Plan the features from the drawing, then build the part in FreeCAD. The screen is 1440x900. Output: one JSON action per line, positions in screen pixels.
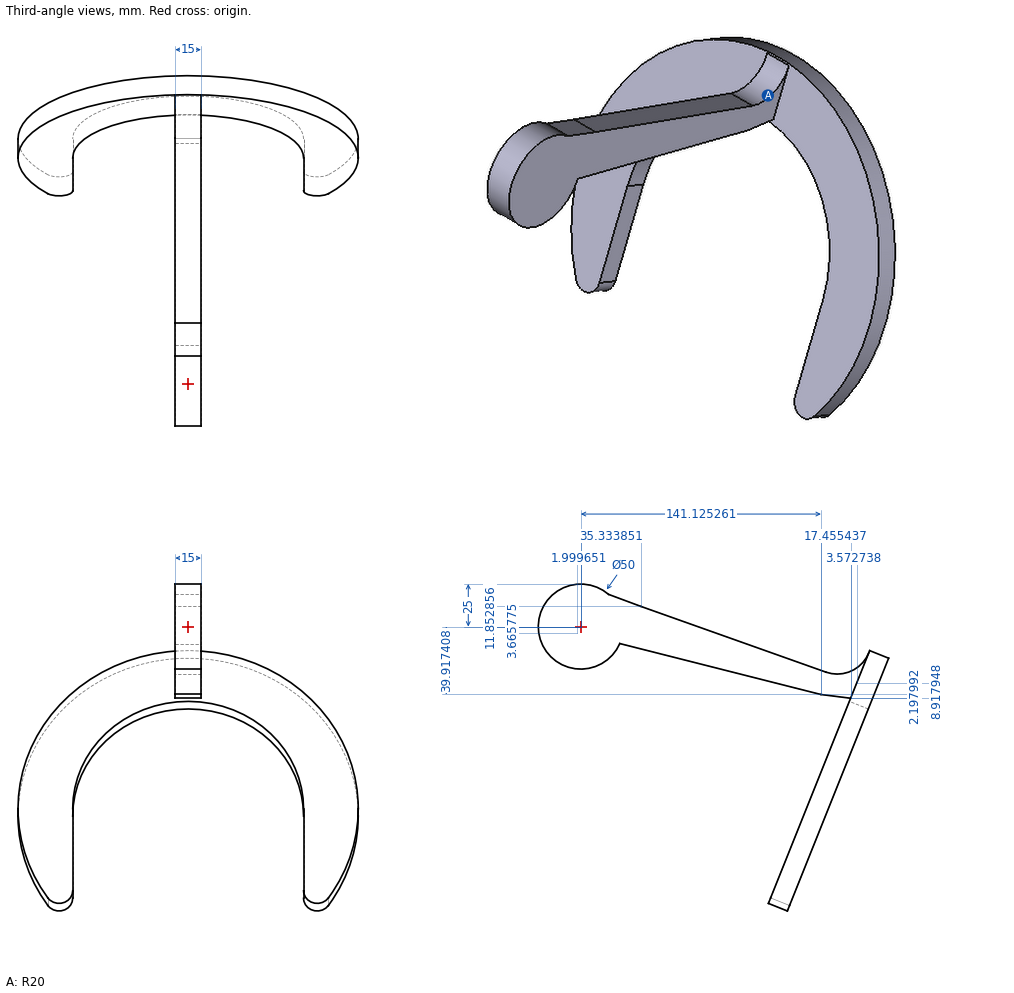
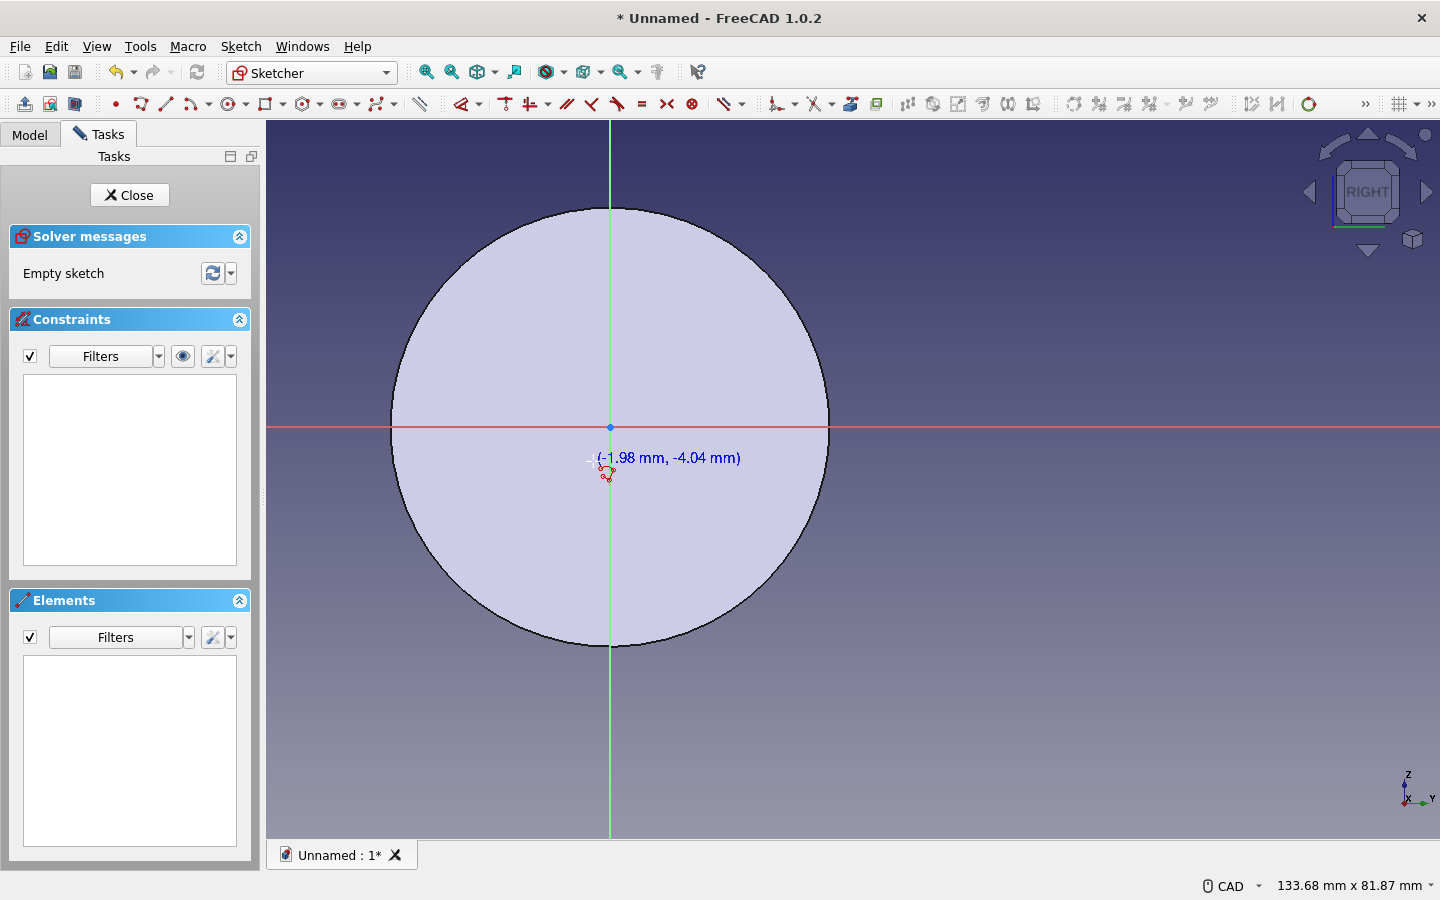
{"action": "left_click", "coordinate": [592, 459]}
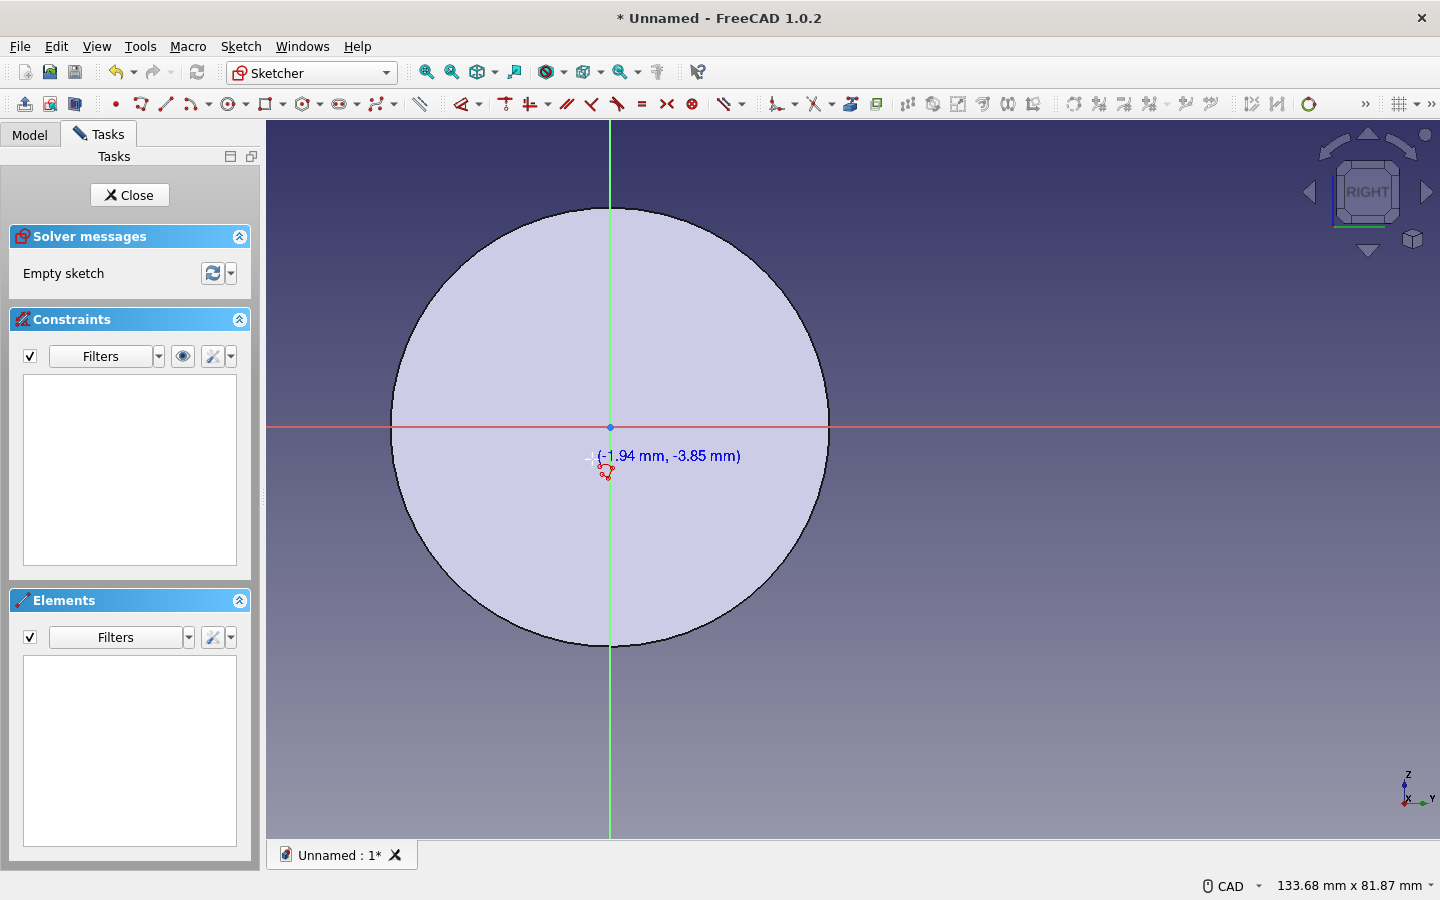
{"action": "scroll", "coordinate": [353, 461], "scroll_direction": "down", "scroll_amount": 4}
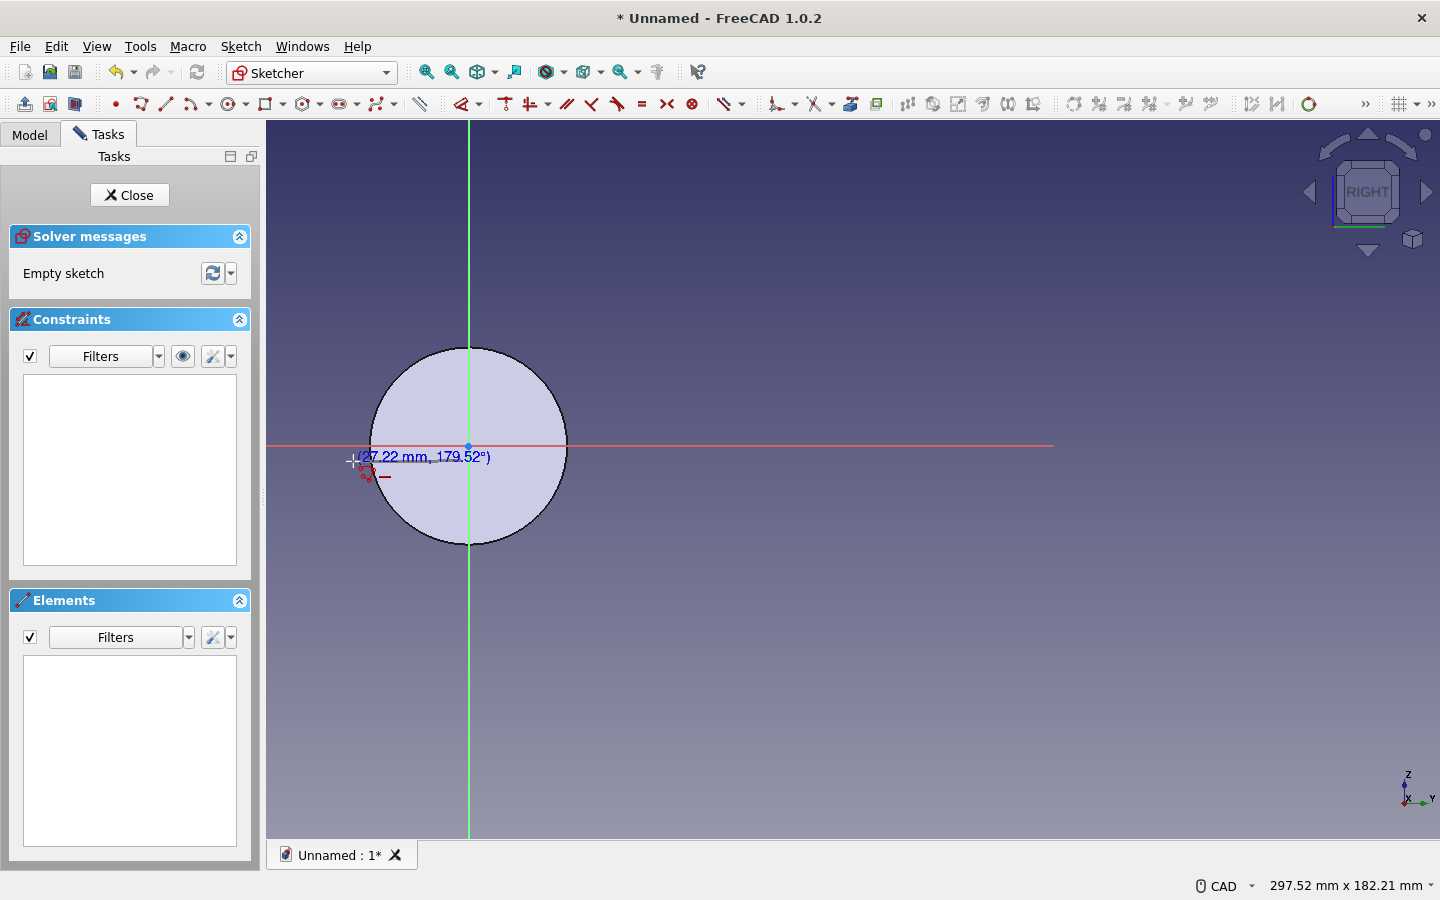
{"action": "left_click", "coordinate": [1025, 604]}
{"action": "left_click", "coordinate": [1094, 612]}
{"action": "left_click", "coordinate": [1108, 577]}
{"action": "left_click", "coordinate": [608, 399]}
{"action": "left_click", "coordinate": [469, 347]}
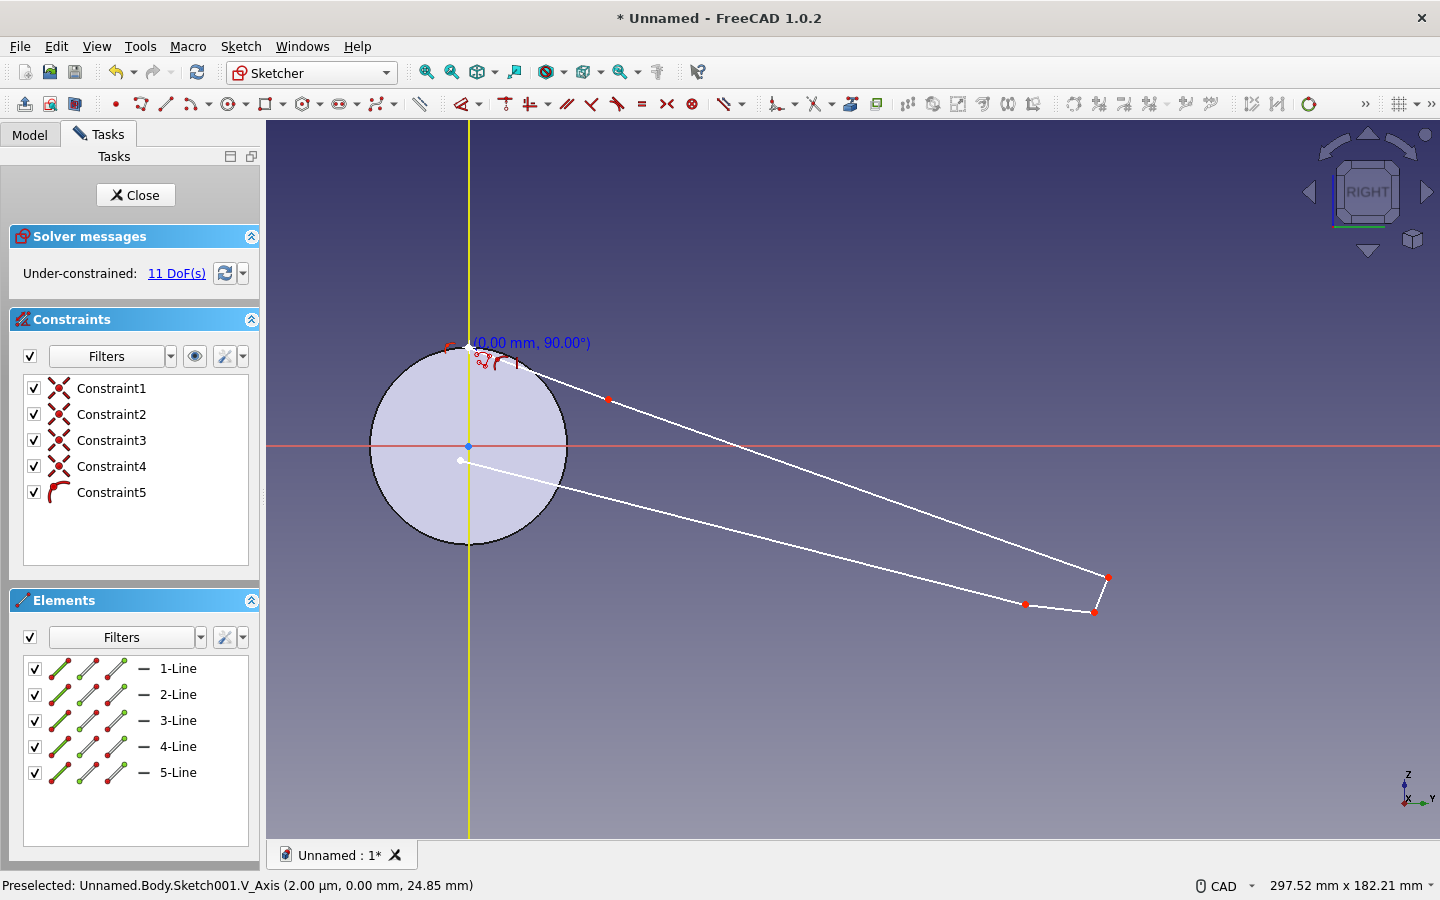
{"action": "scroll", "coordinate": [461, 461], "scroll_direction": "up", "scroll_amount": 4}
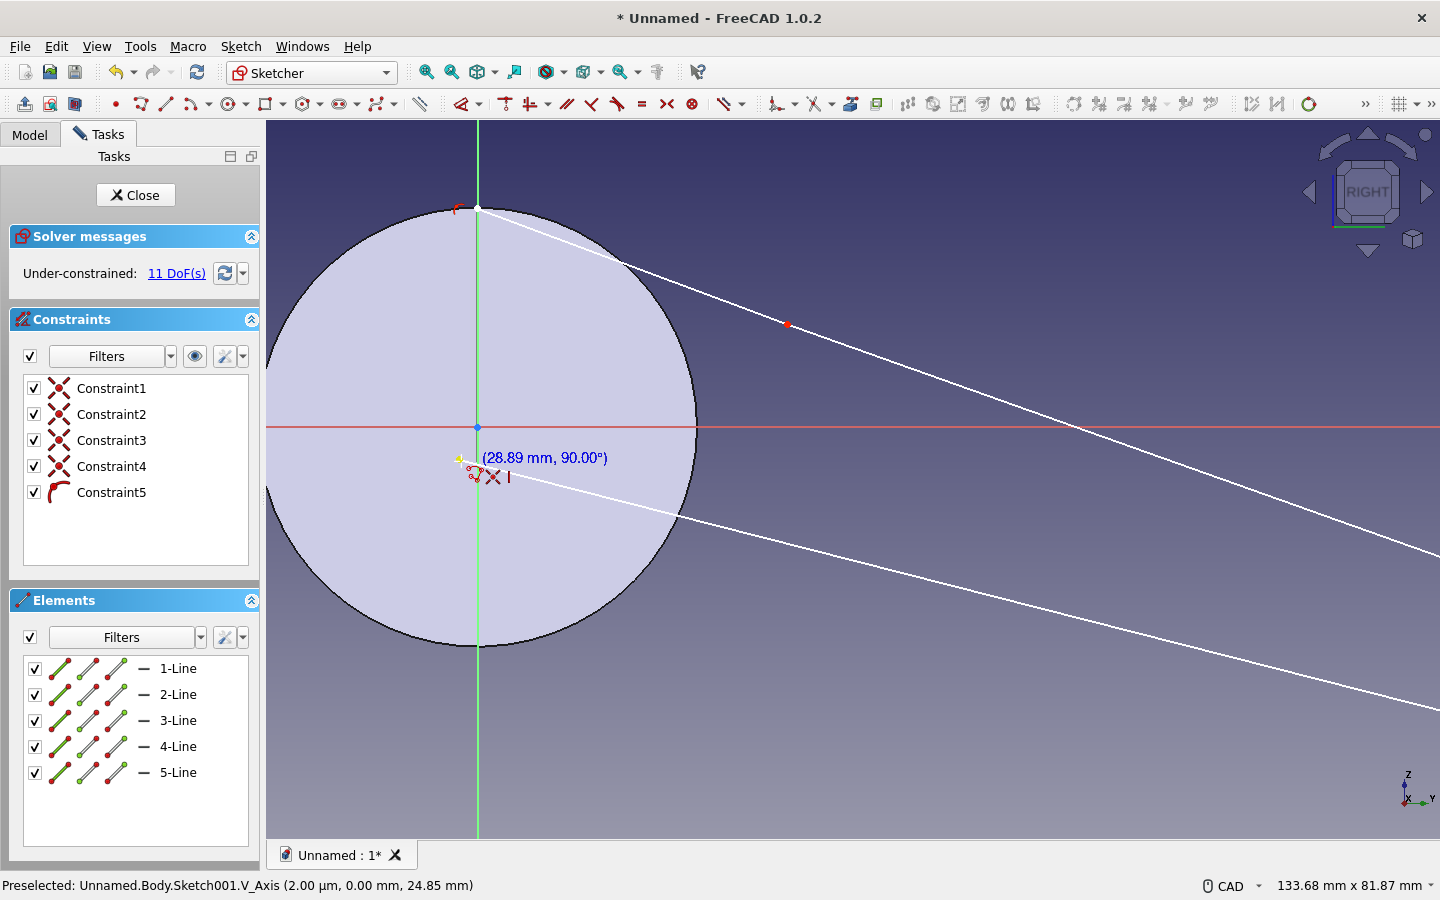
{"action": "left_click", "coordinate": [460, 460]}
{"action": "key", "text": "Escape"}
{"action": "key", "text": "Escape"}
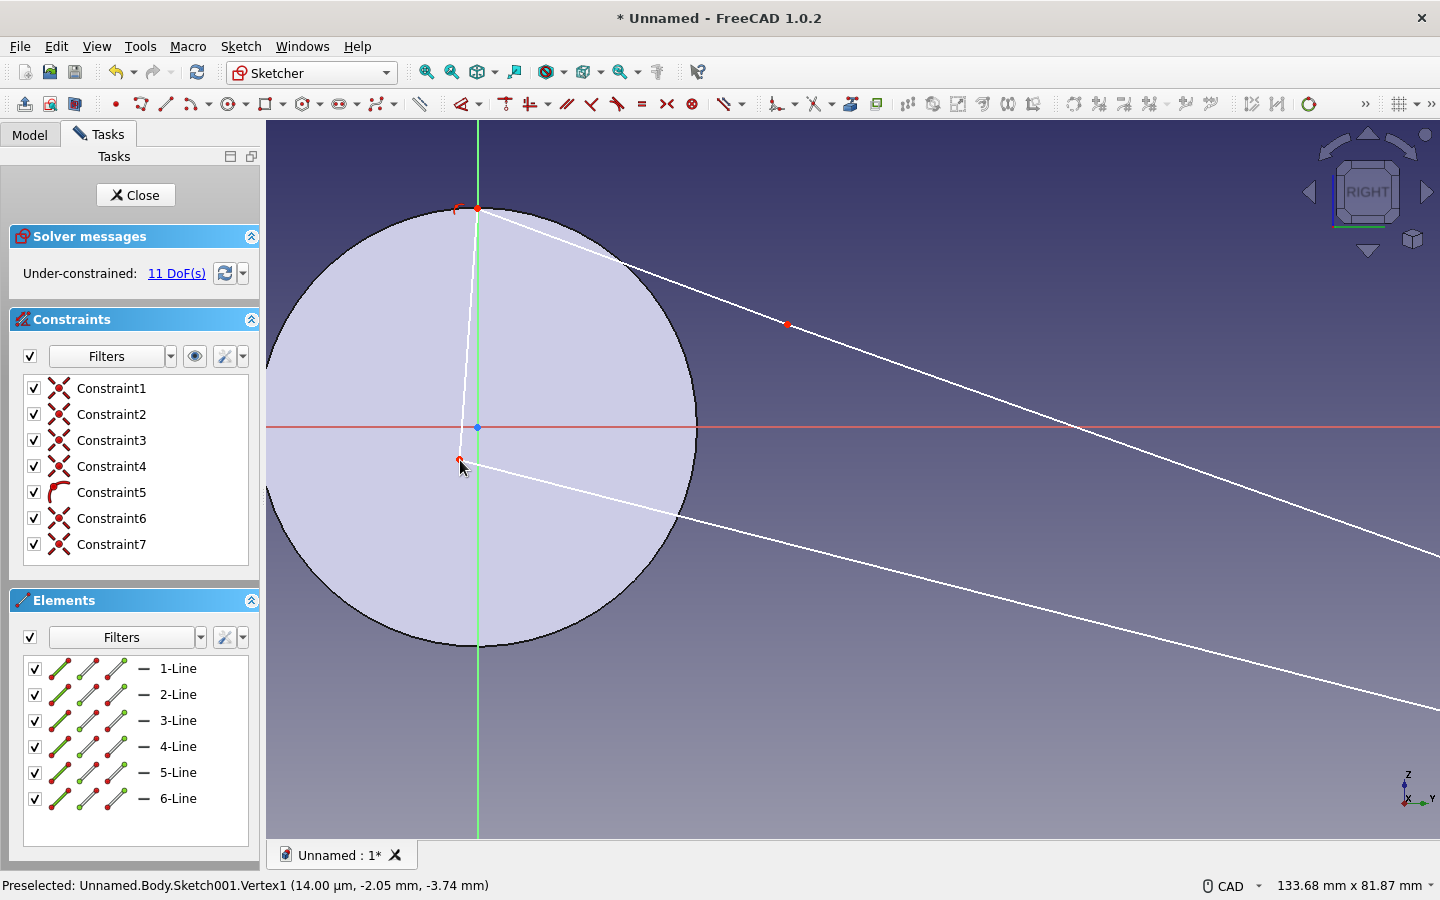
{"action": "key", "text": "d"}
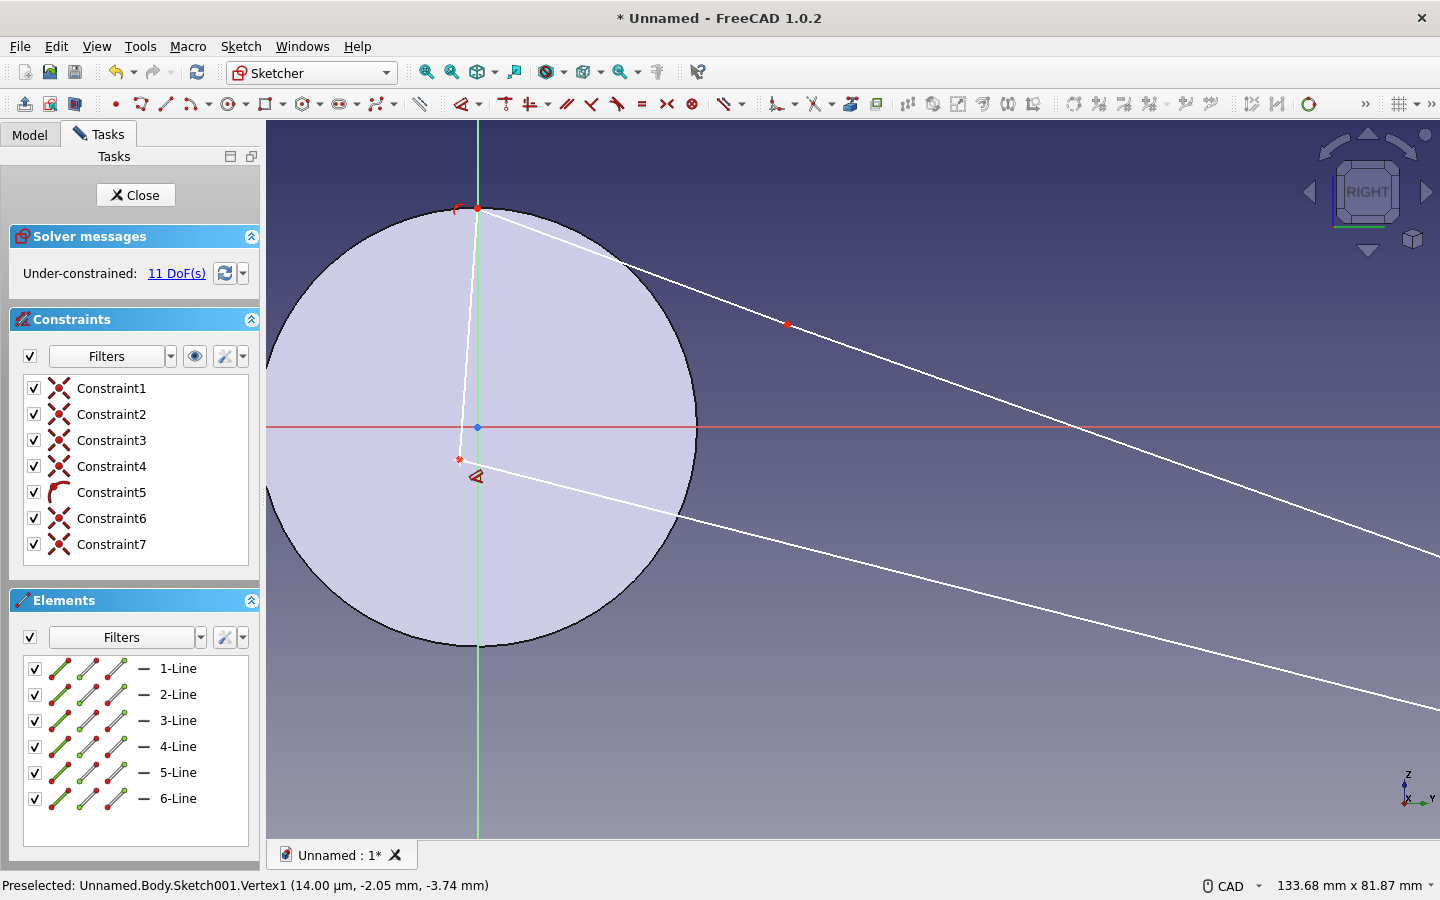
{"action": "left_click", "coordinate": [478, 209]}
{"action": "left_click", "coordinate": [444, 318]}